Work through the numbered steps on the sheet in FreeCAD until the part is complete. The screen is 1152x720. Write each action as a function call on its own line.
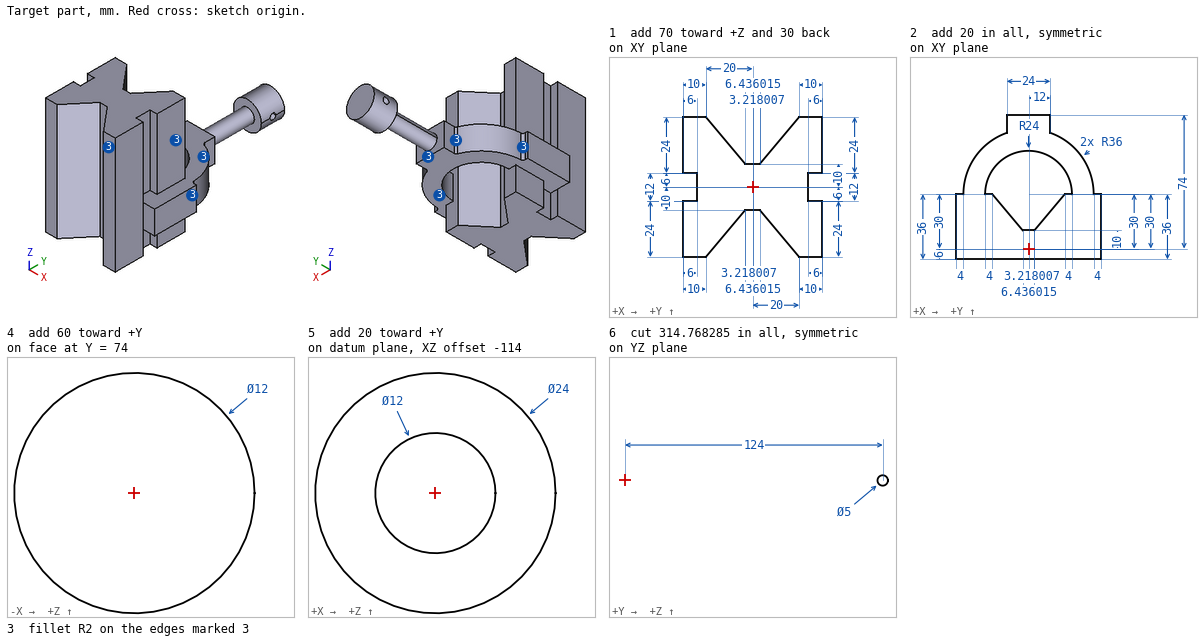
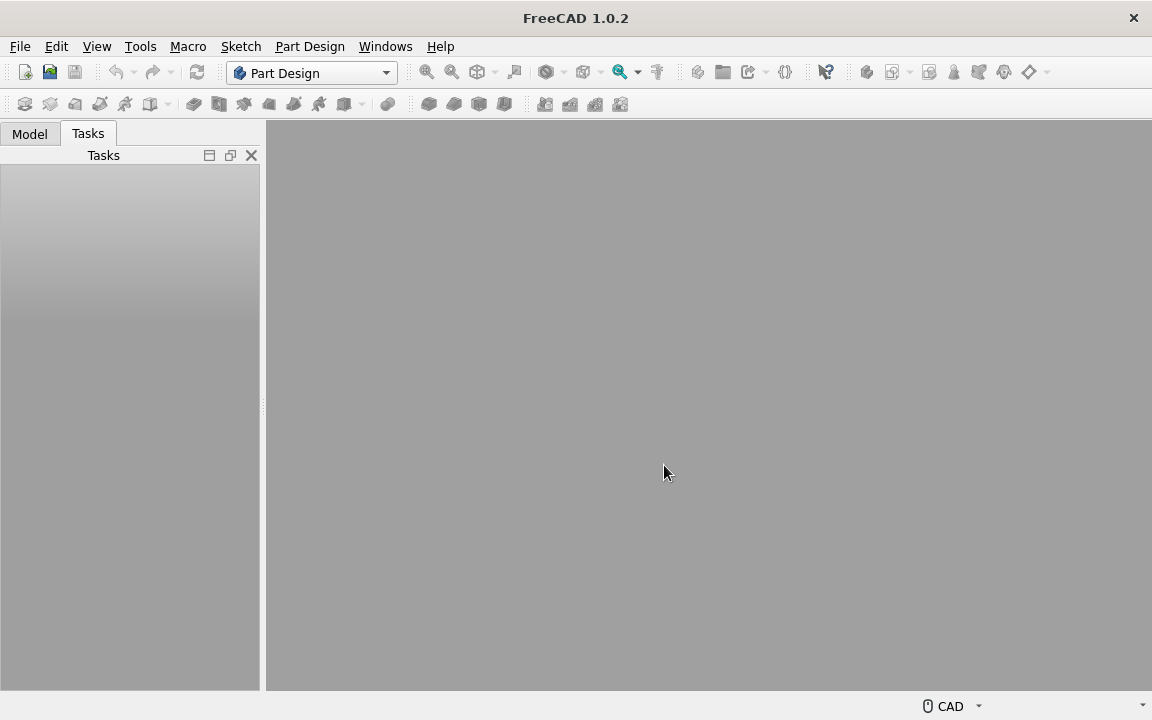
click(25, 72)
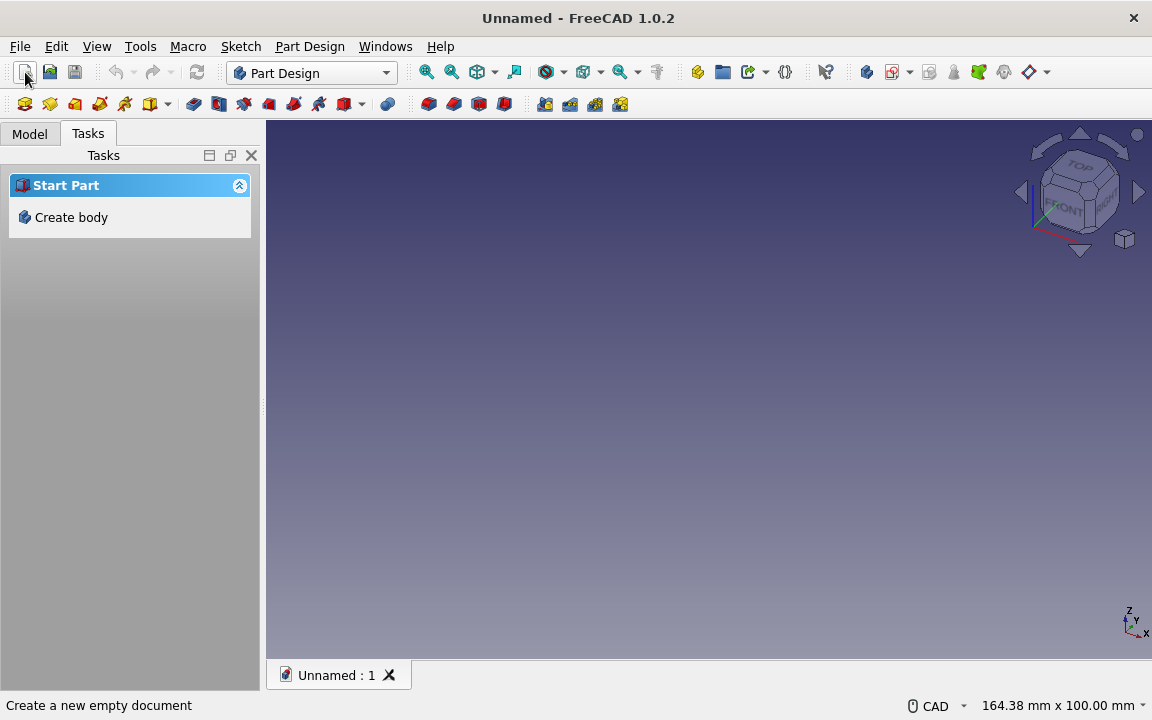
click(892, 72)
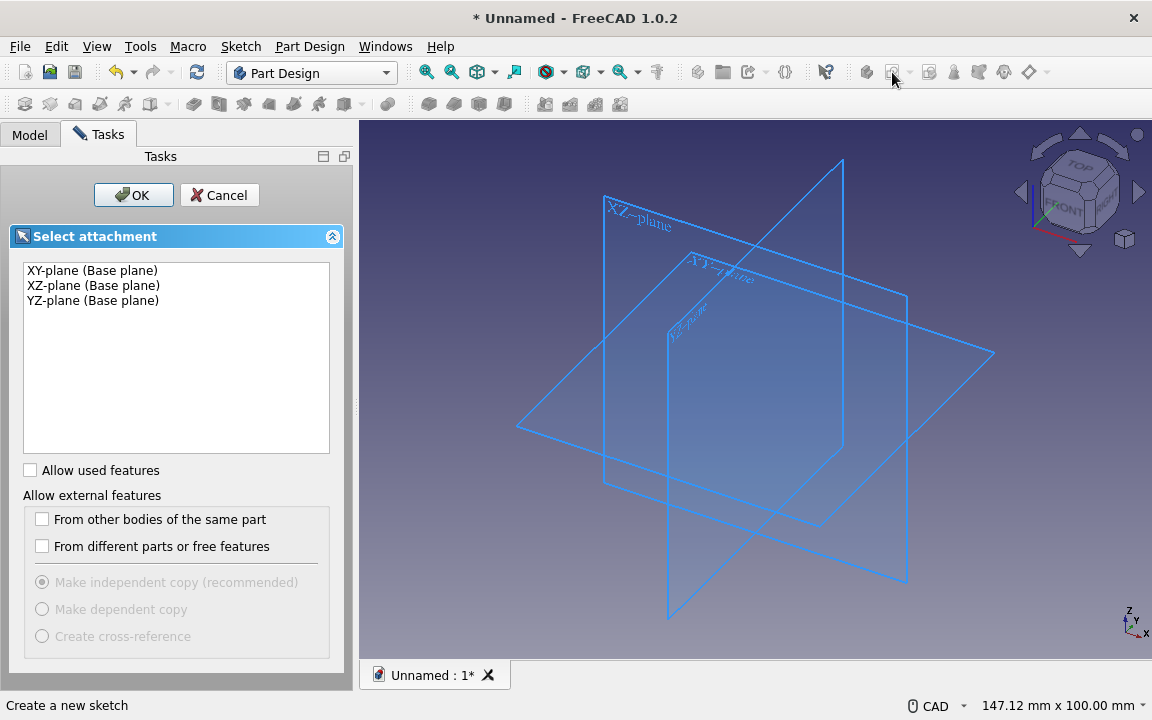
click(84, 270)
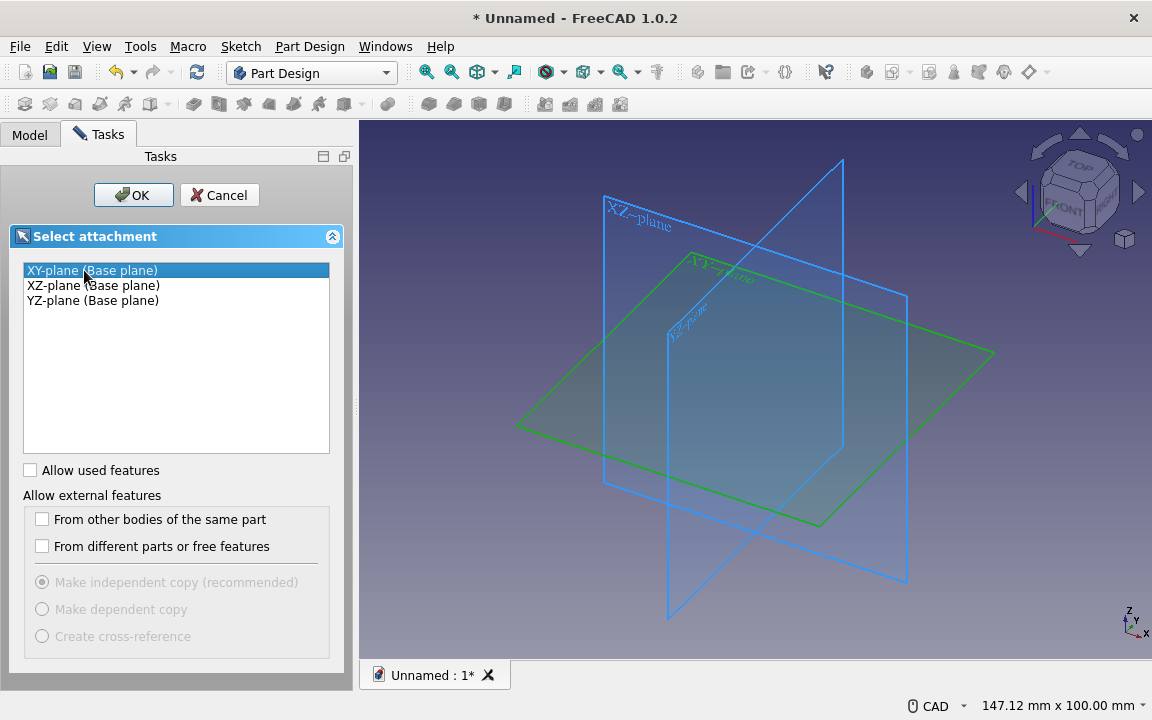
click(134, 195)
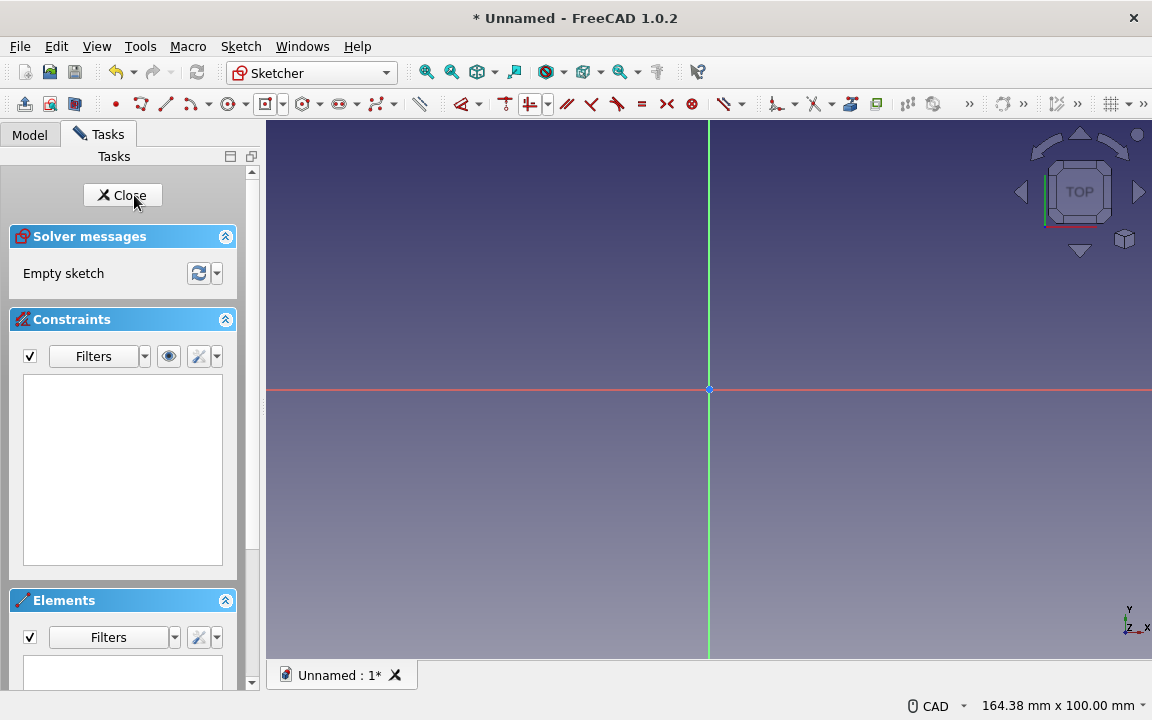
click(141, 104)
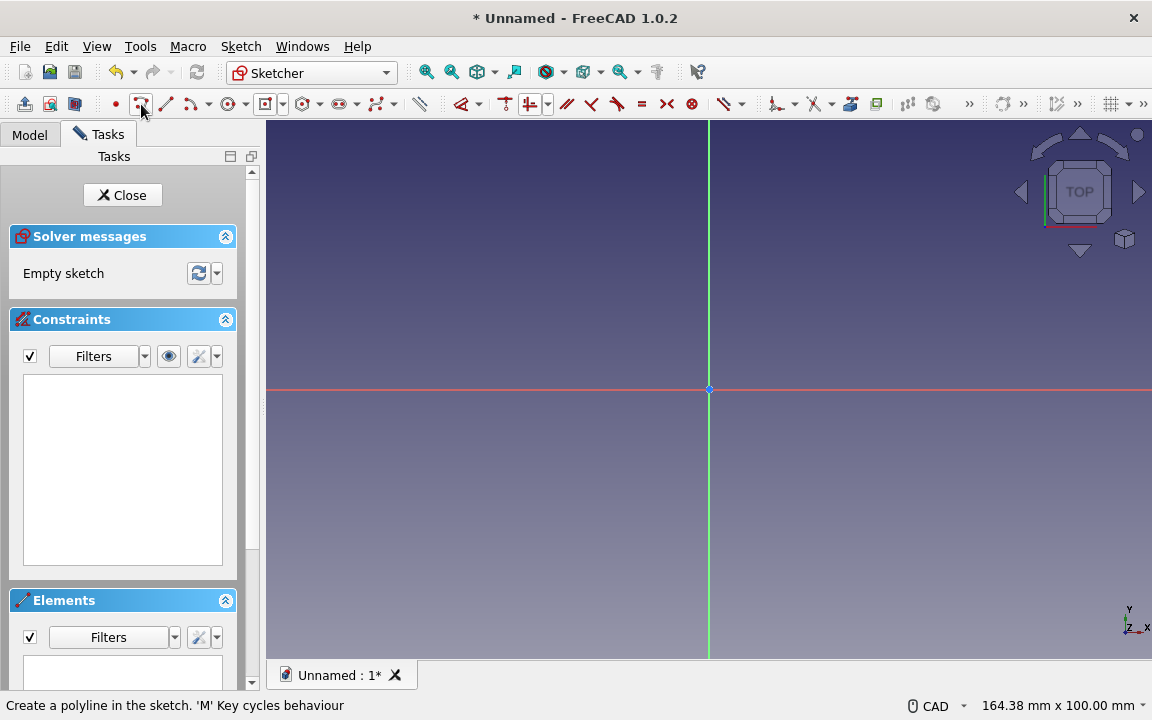
click(692, 443)
click(726, 443)
click(817, 551)
click(871, 551)
click(871, 422)
click(838, 422)
click(838, 357)
click(871, 357)
click(871, 228)
click(817, 228)
click(726, 336)
click(692, 336)
click(601, 228)
click(547, 228)
click(547, 357)
click(580, 357)
click(580, 422)
click(547, 422)
click(547, 551)
click(601, 551)
click(692, 444)
key(Escape)
key(Escape)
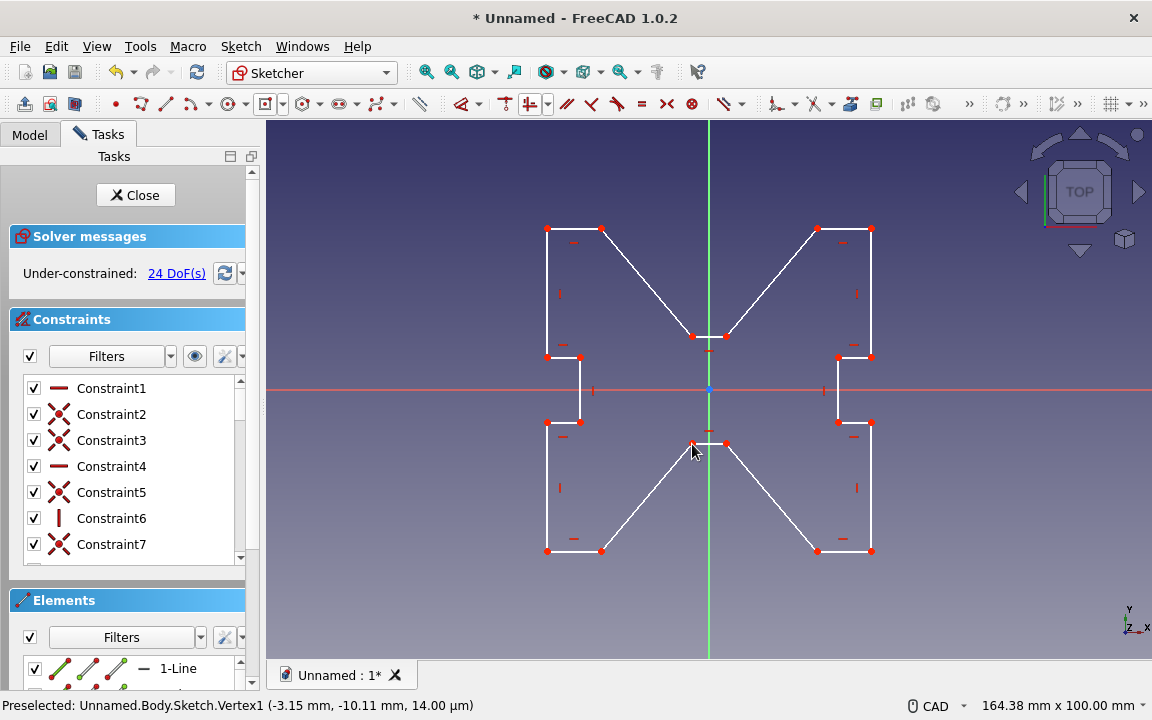
click(460, 104)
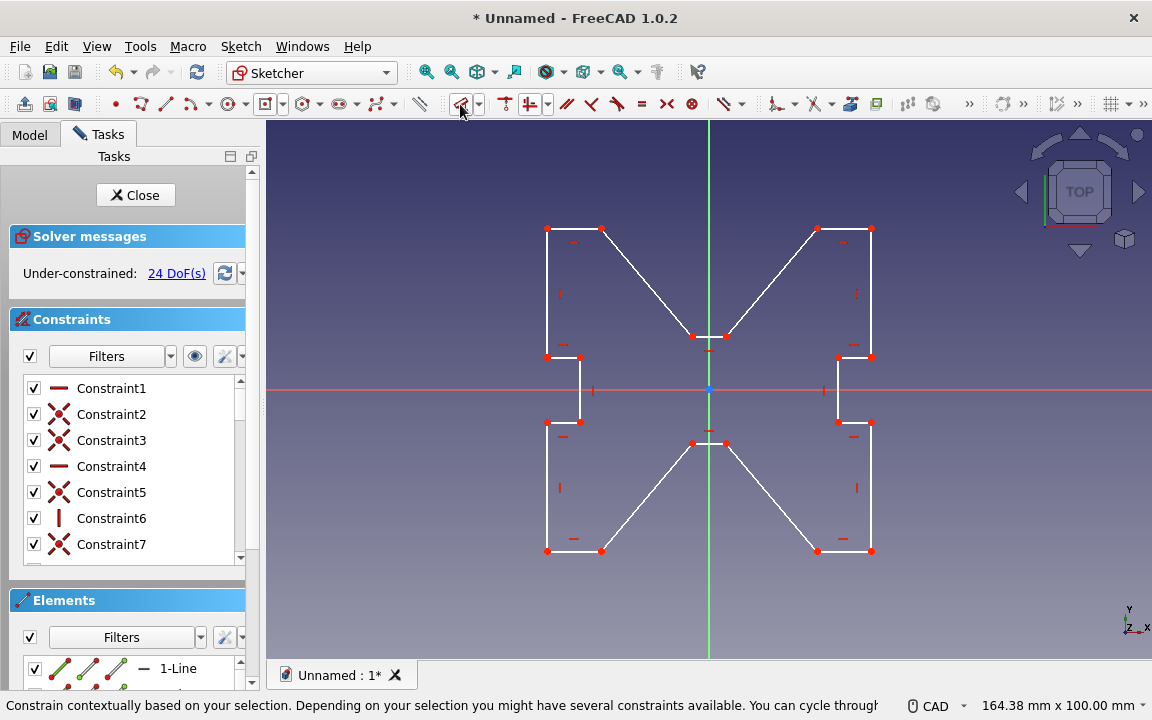
scroll(861, 423, up, 2)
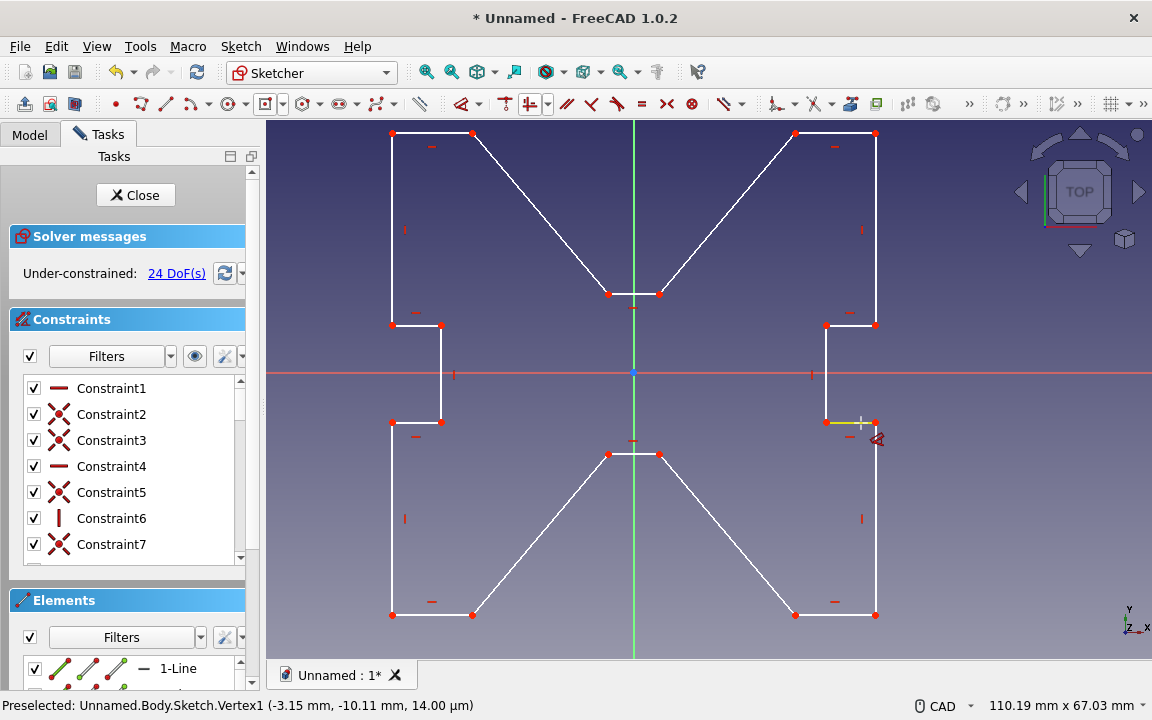
click(861, 423)
click(851, 457)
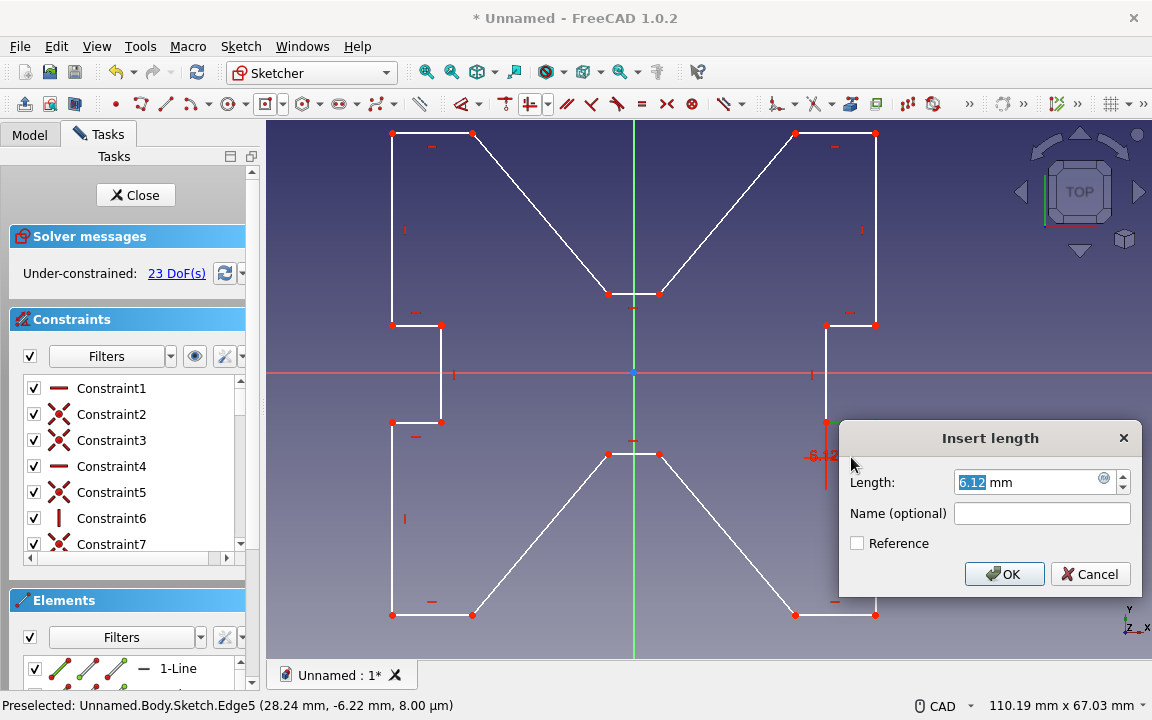
text(6)
key(Return)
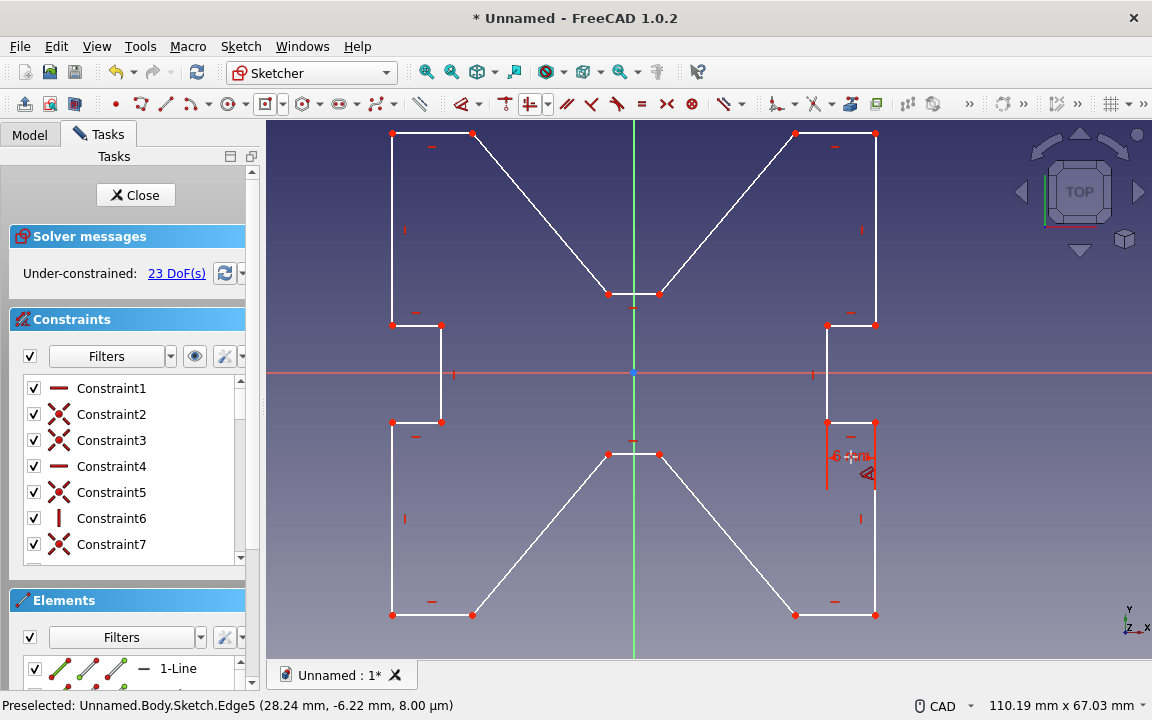
click(842, 326)
click(851, 292)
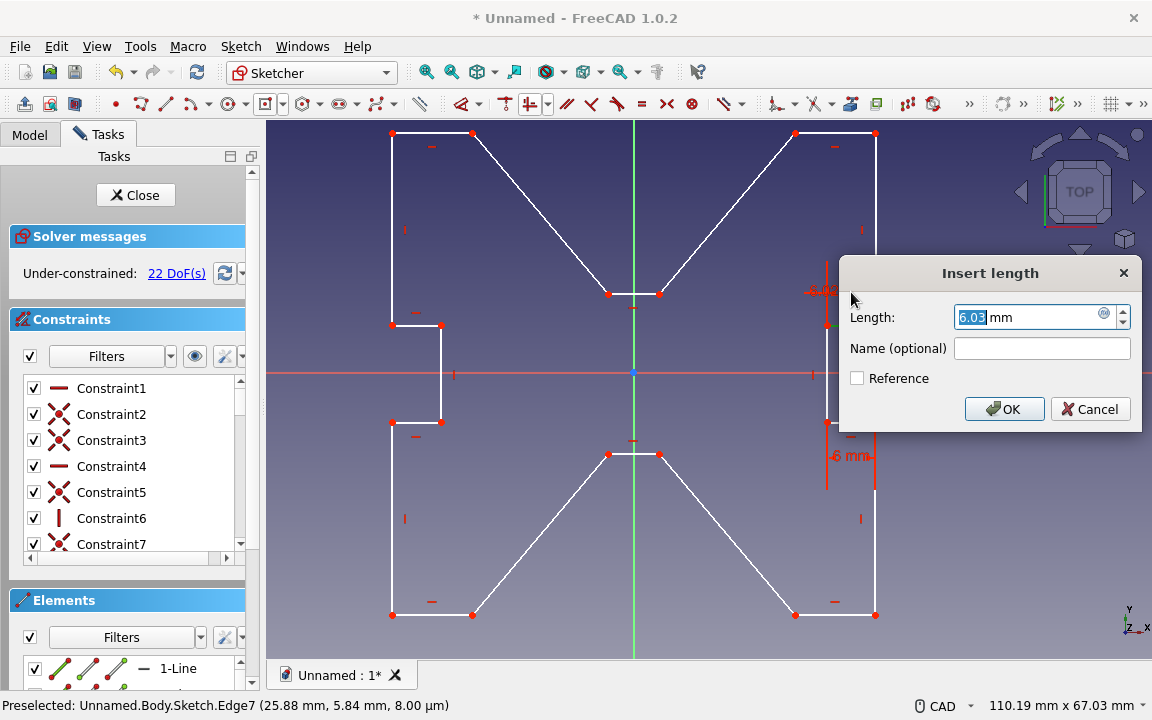
text(6)
key(Return)